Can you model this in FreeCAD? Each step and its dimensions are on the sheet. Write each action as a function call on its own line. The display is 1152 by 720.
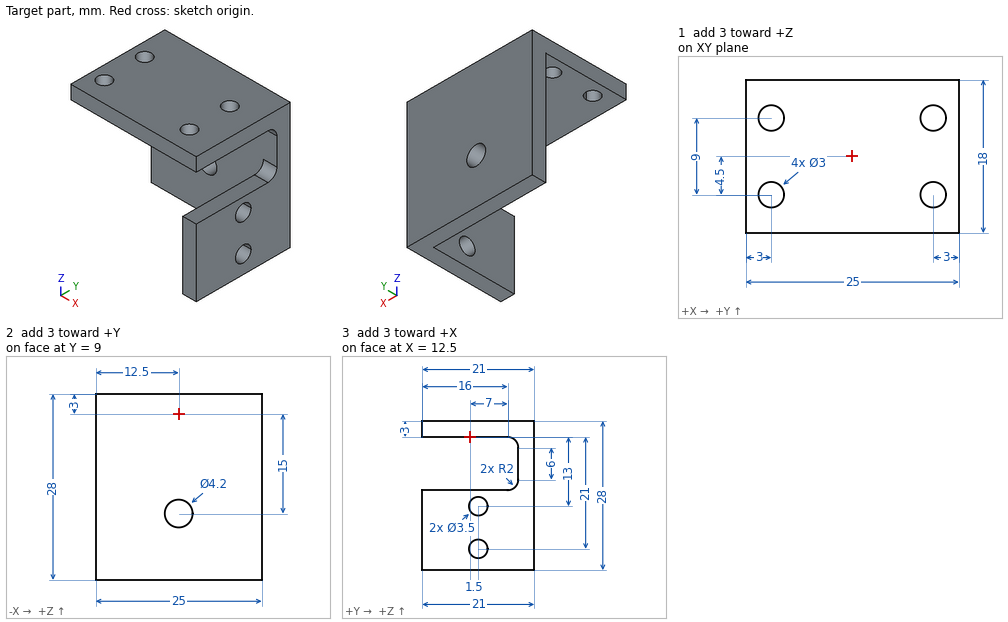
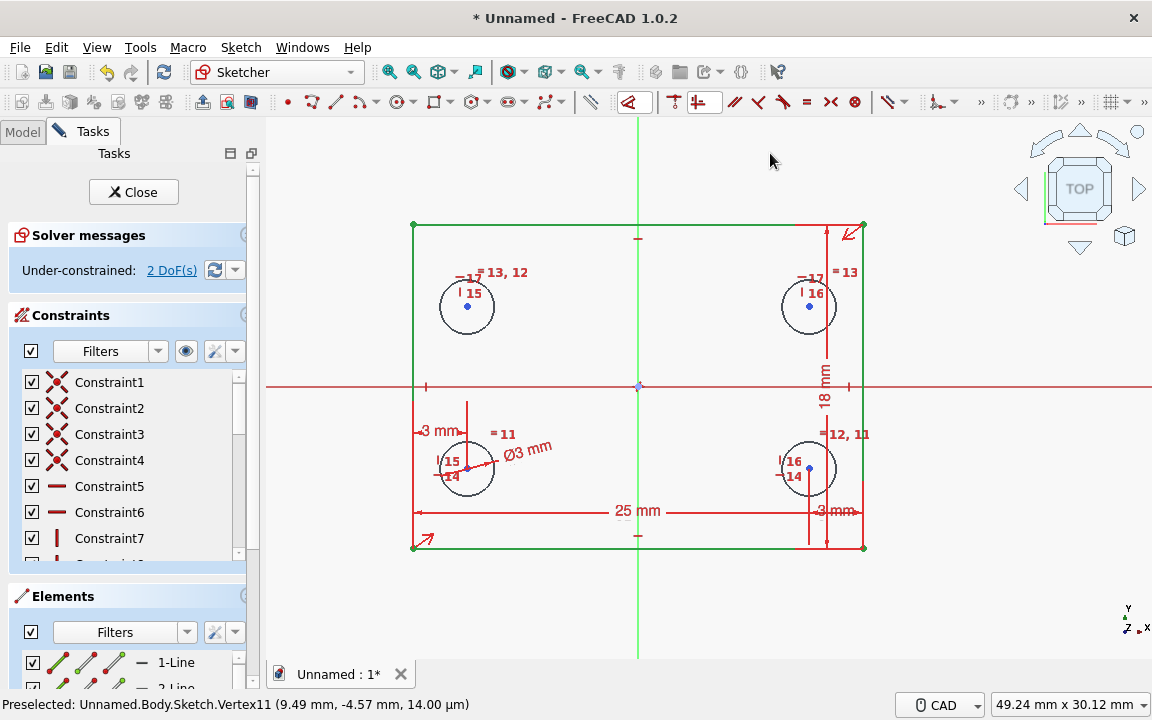
click(467, 469)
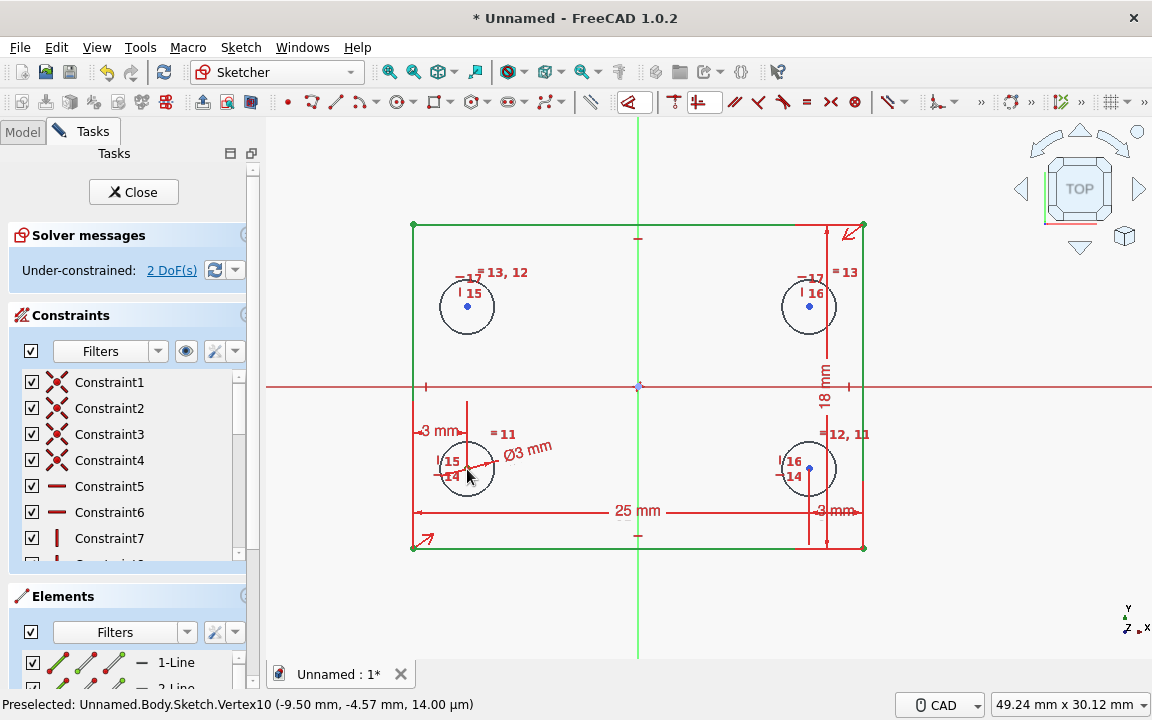
click(467, 307)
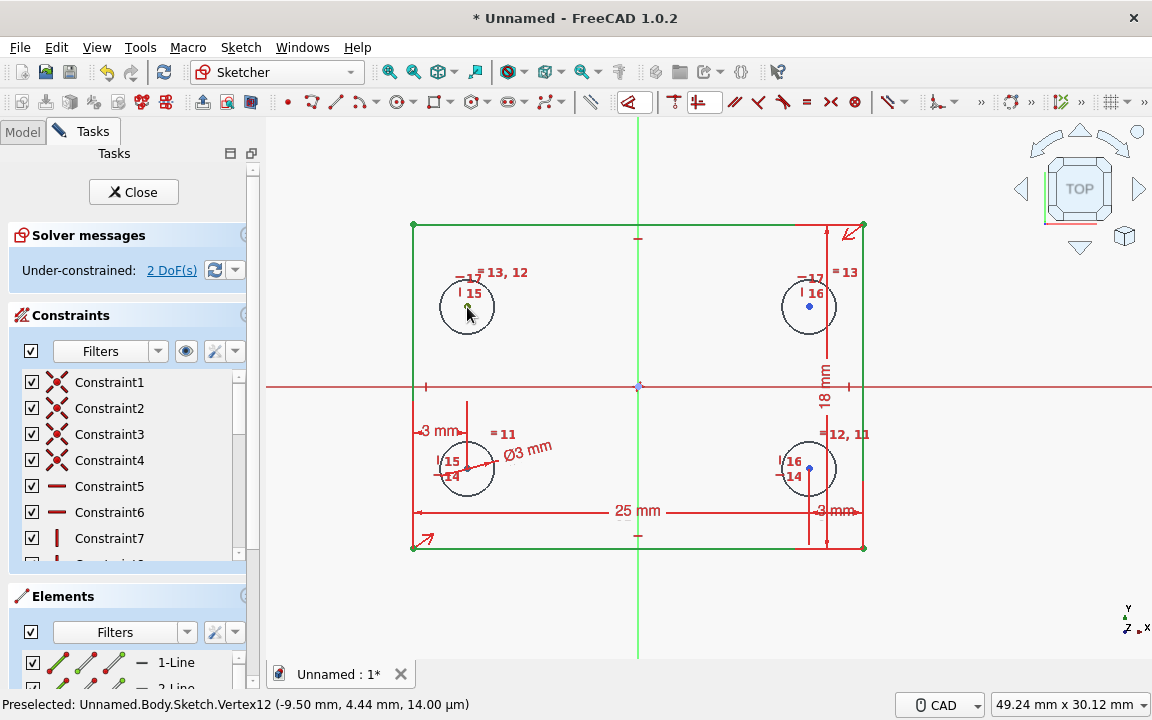
key(i)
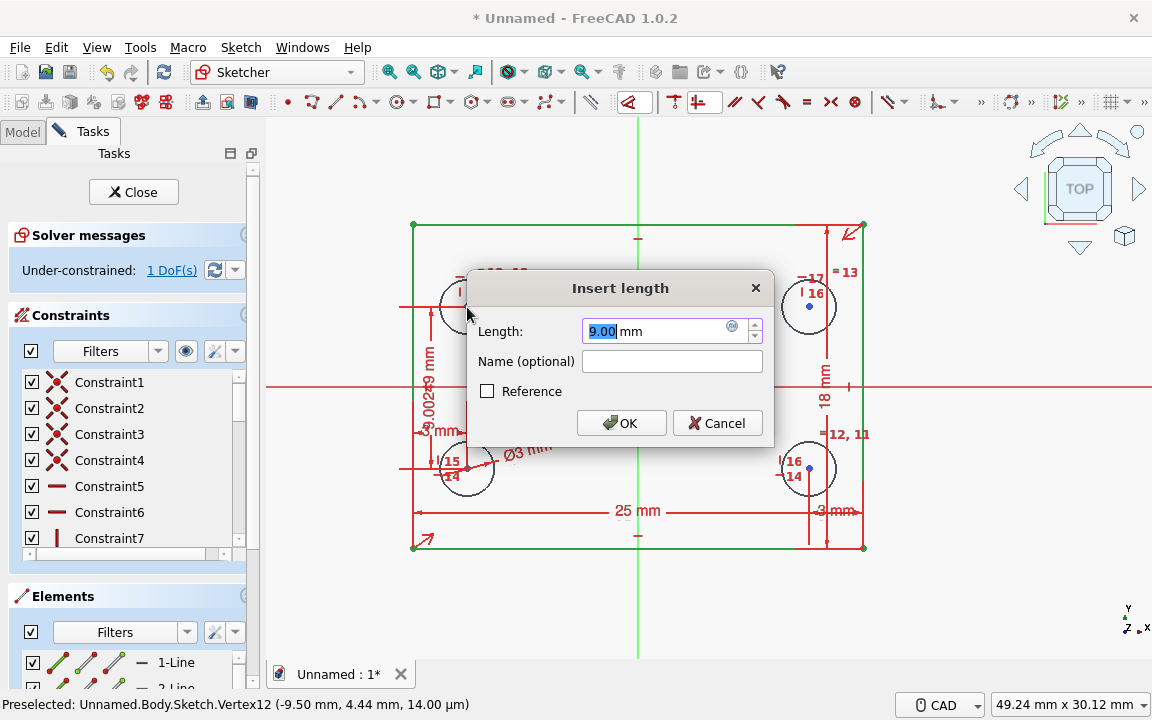
text(9)
key(Return)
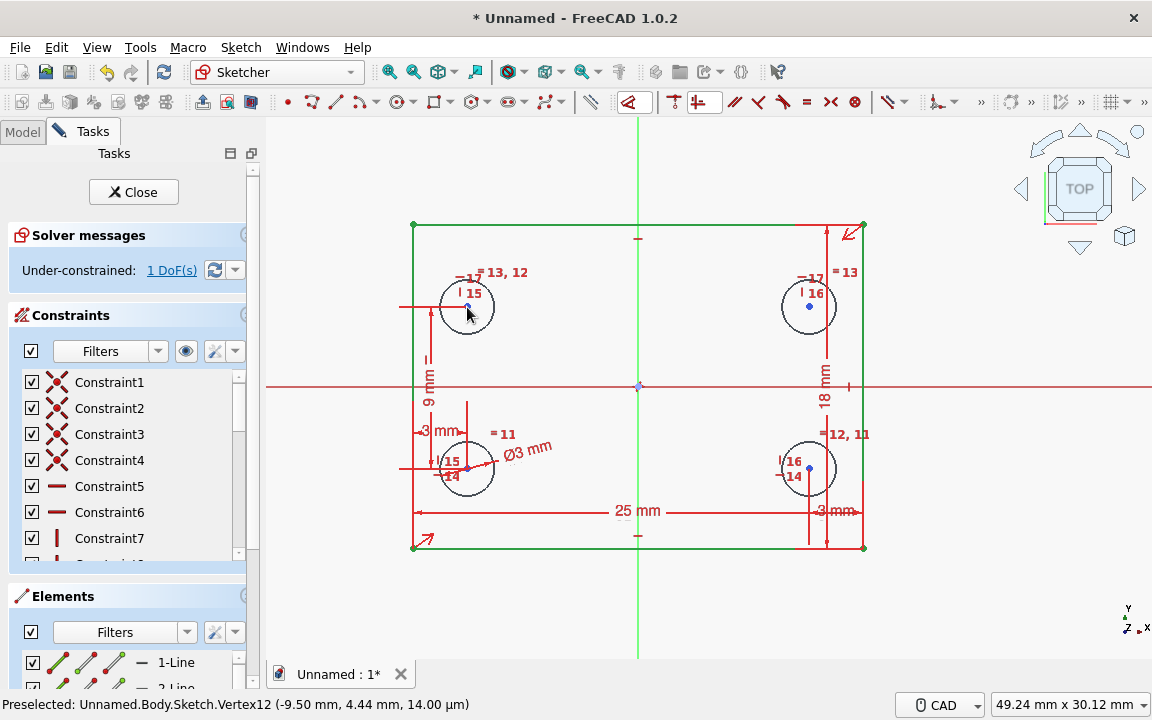
click(467, 469)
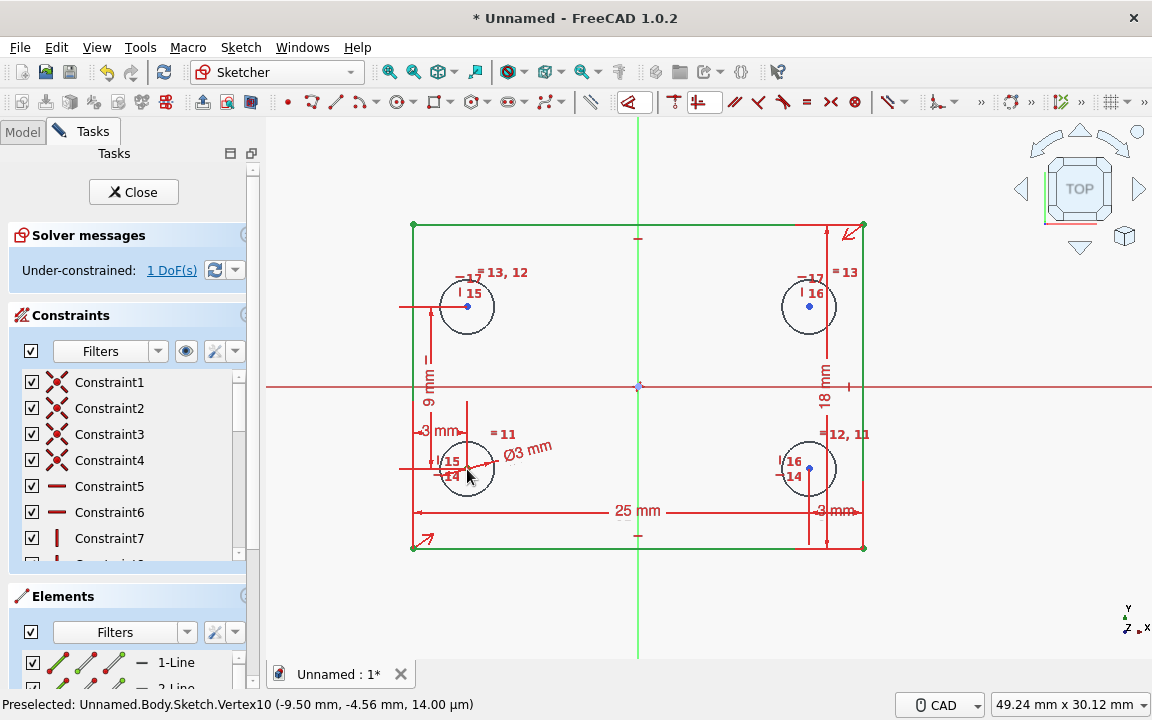
key(i)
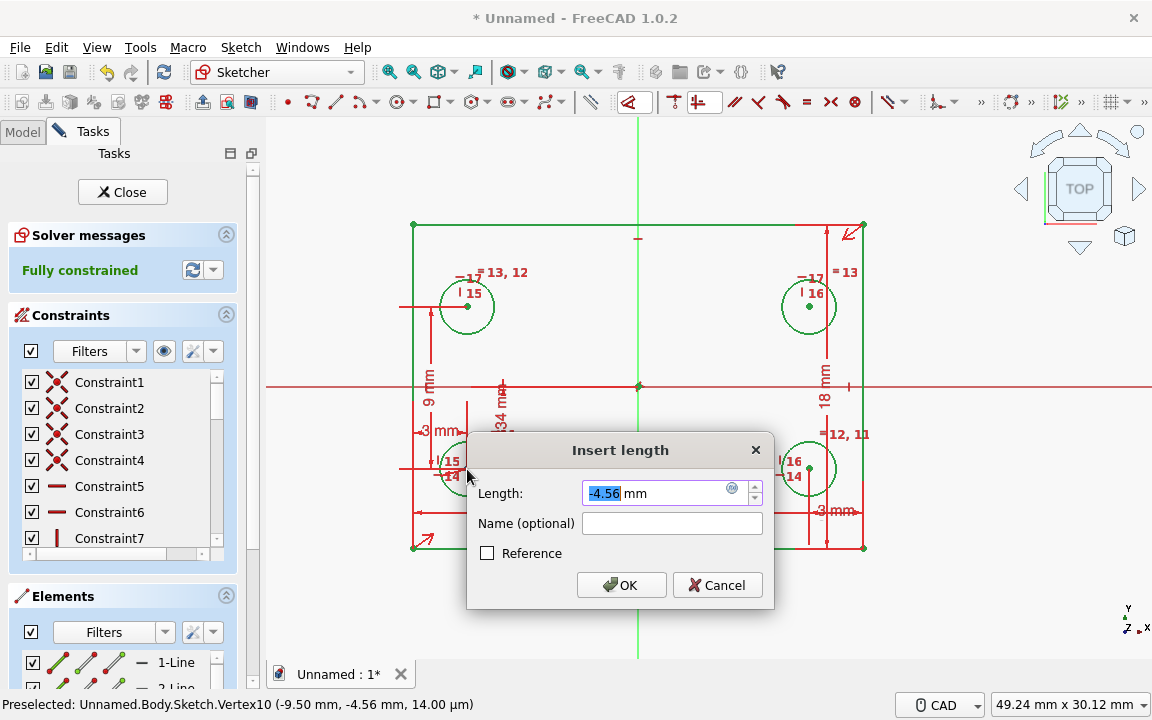
text(-4.5)
key(Return)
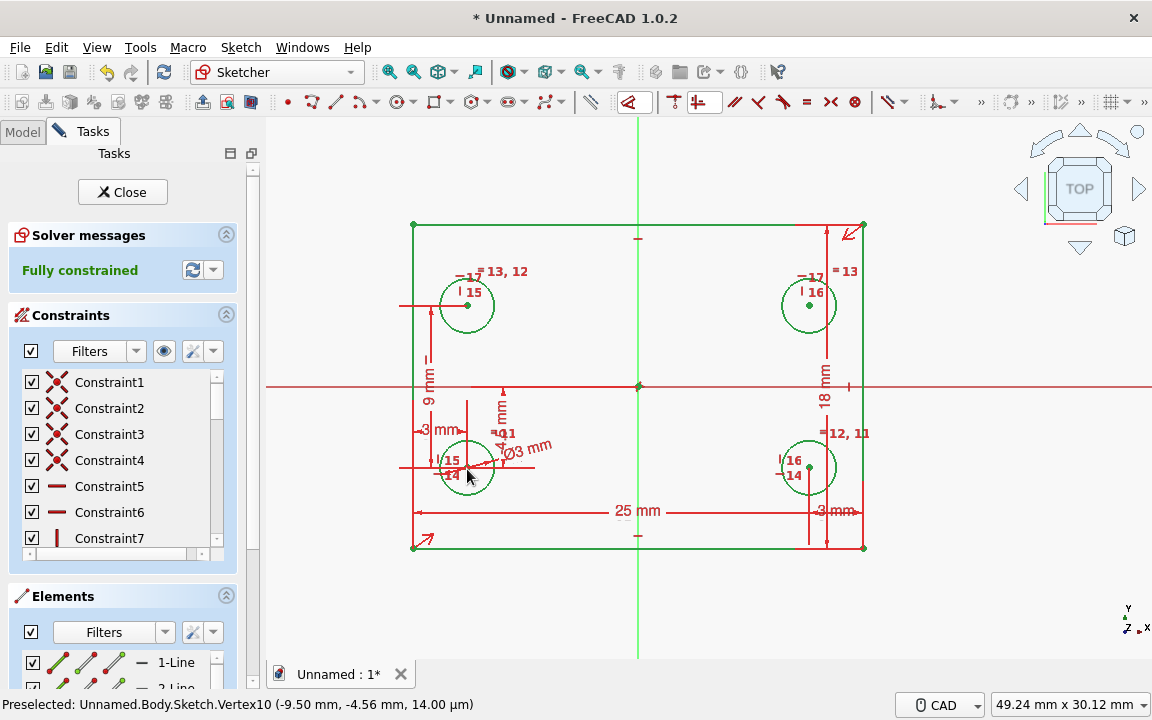
click(123, 192)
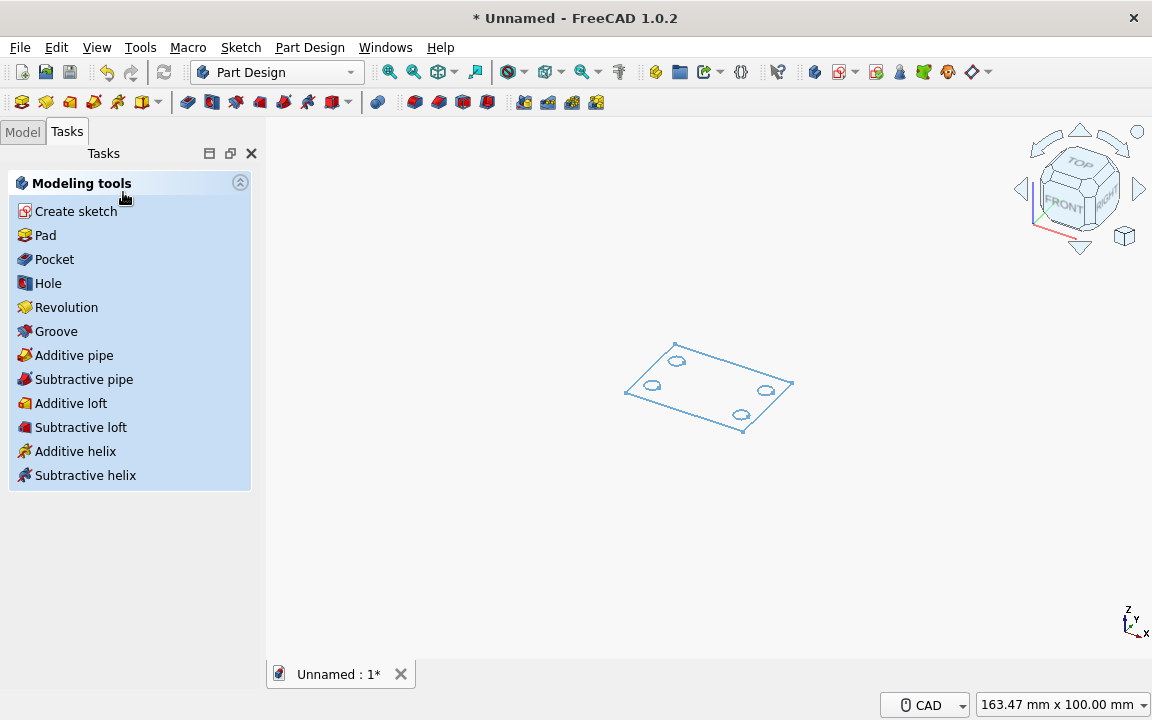
click(22, 102)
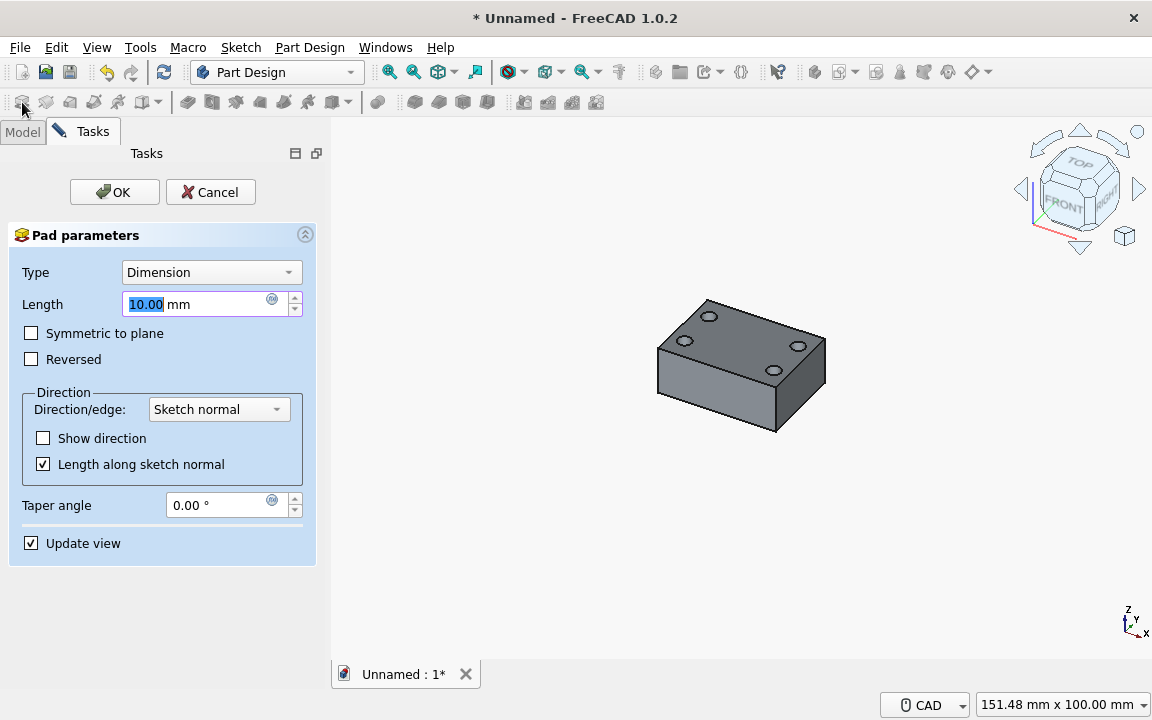
text(3)
key(Tab)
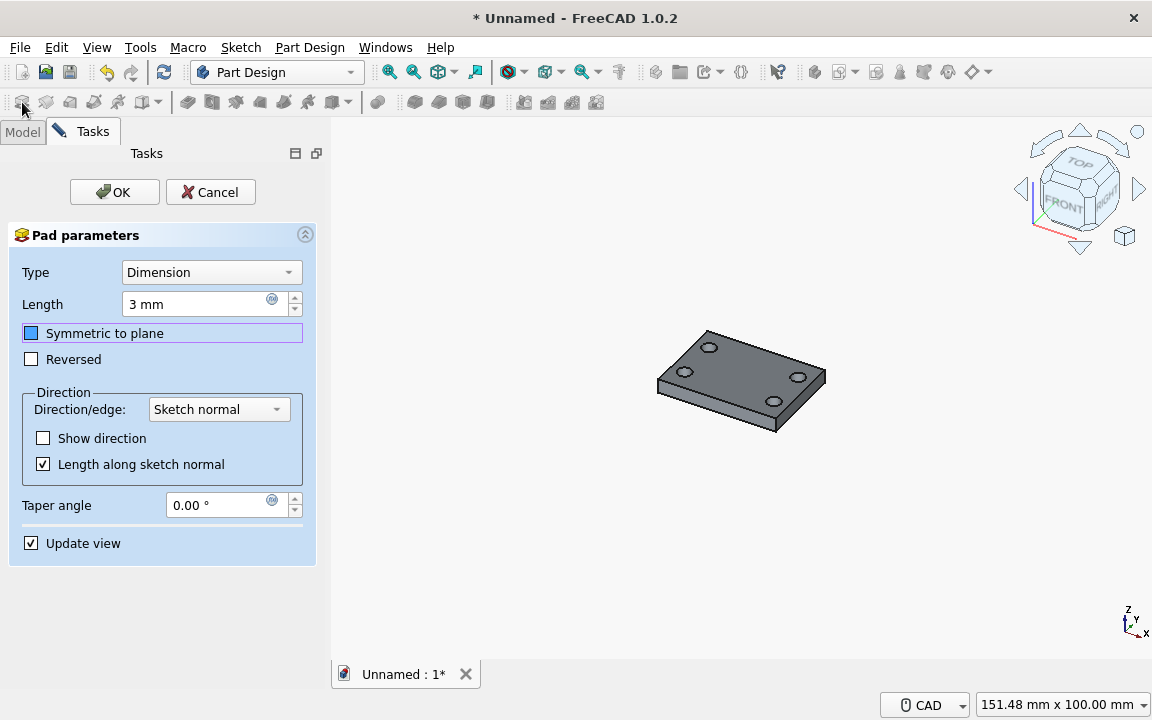
click(115, 192)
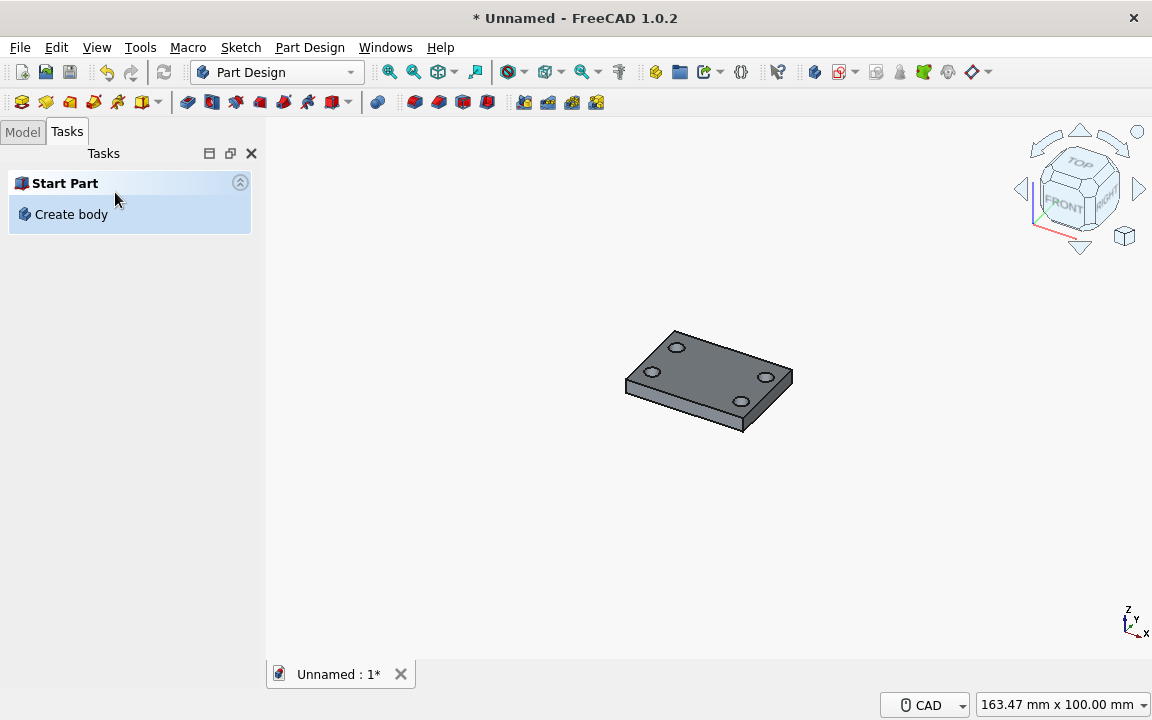
key(v)
key(f)